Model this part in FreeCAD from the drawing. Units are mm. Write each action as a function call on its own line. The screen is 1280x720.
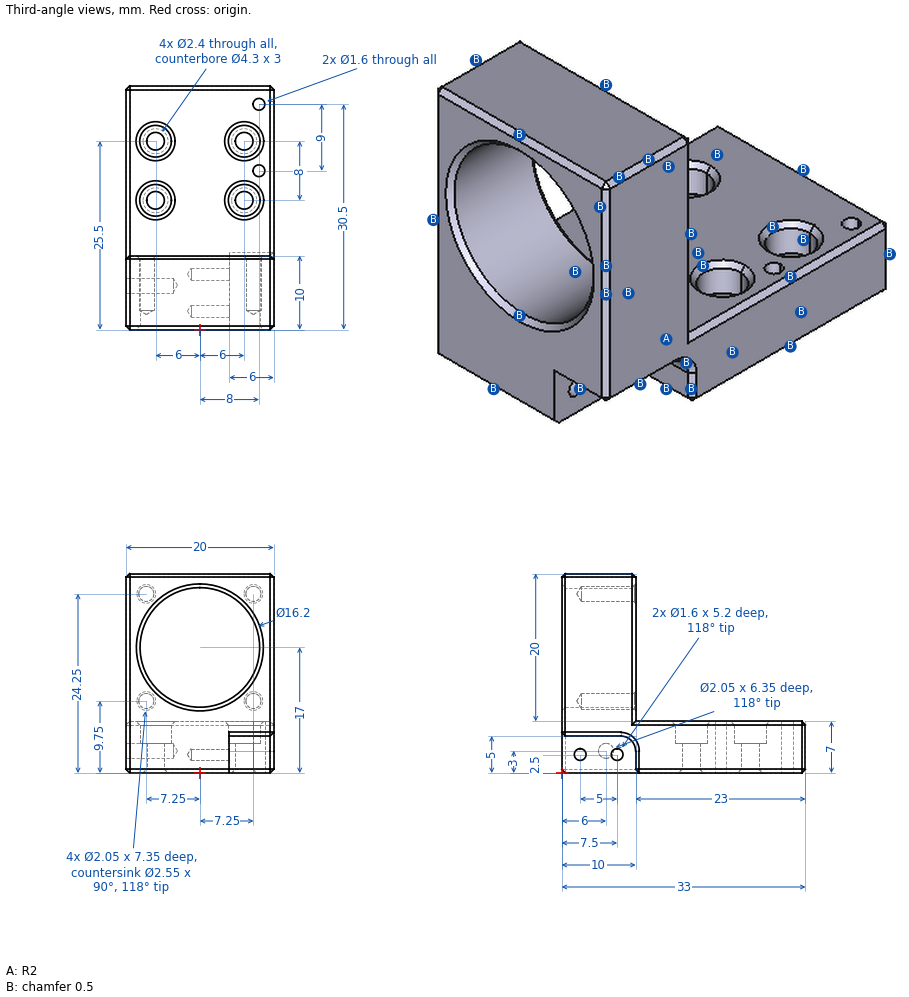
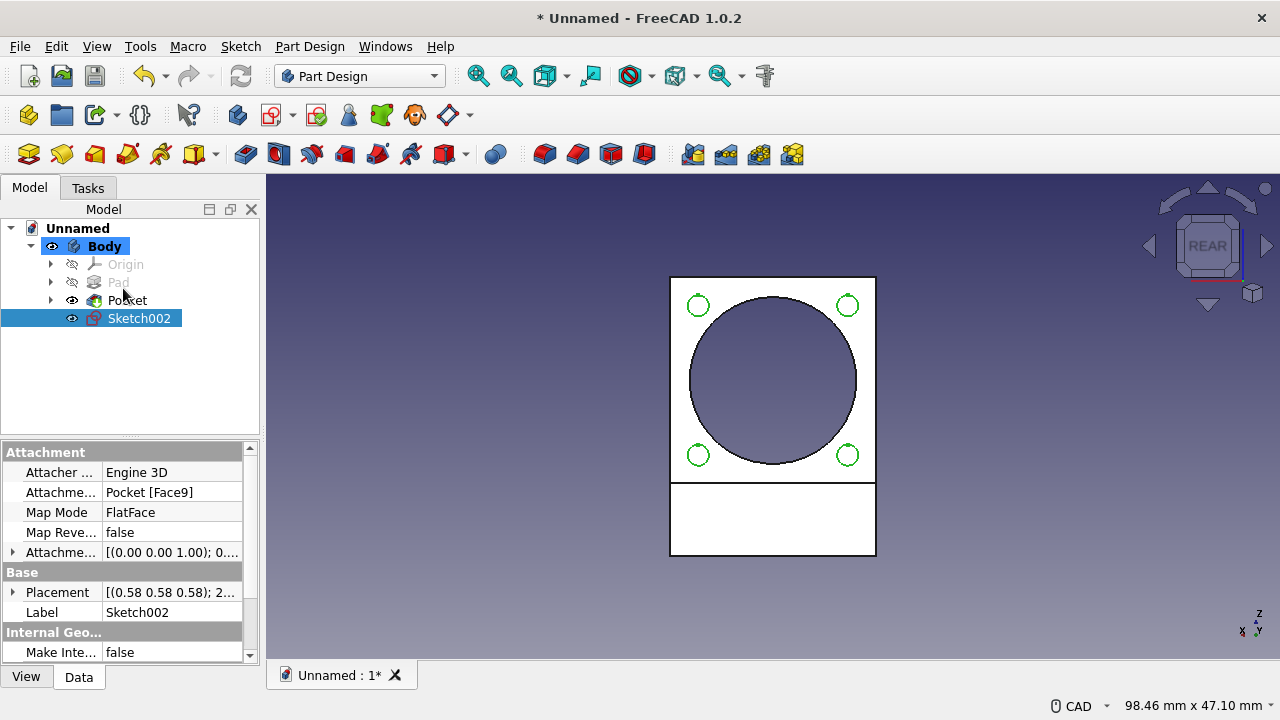
click(279, 154)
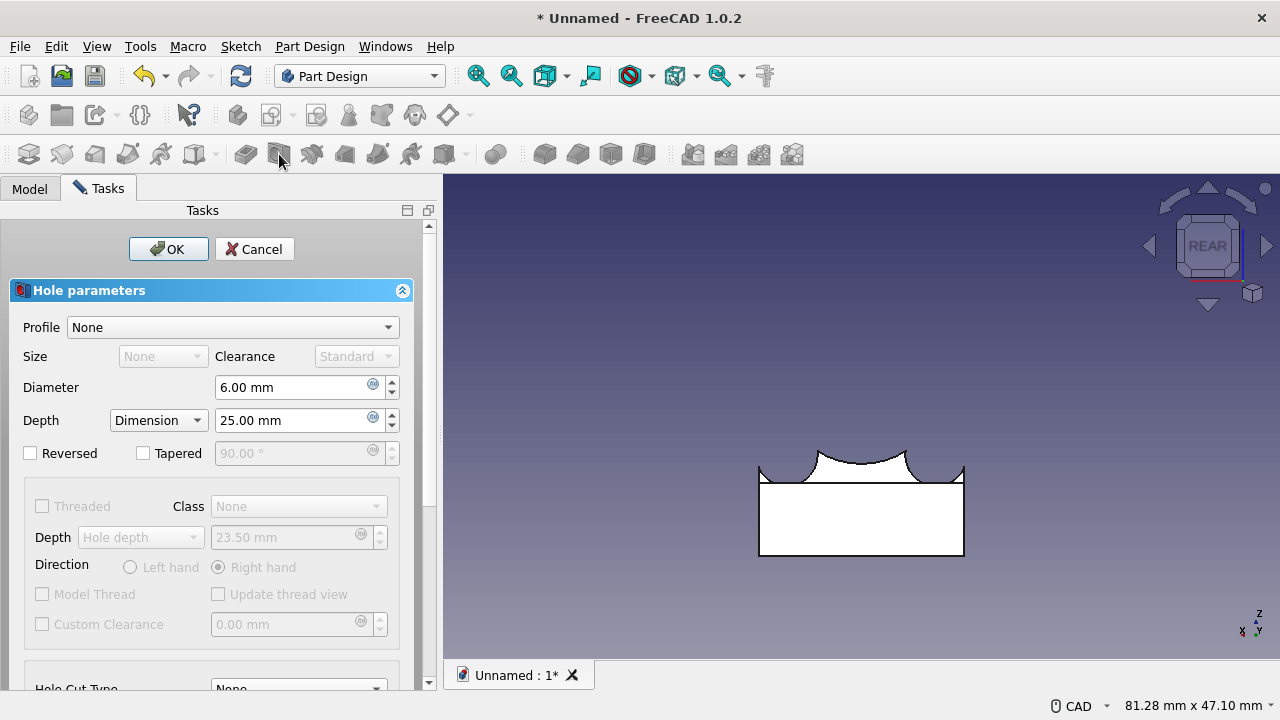
triple_click(300, 388)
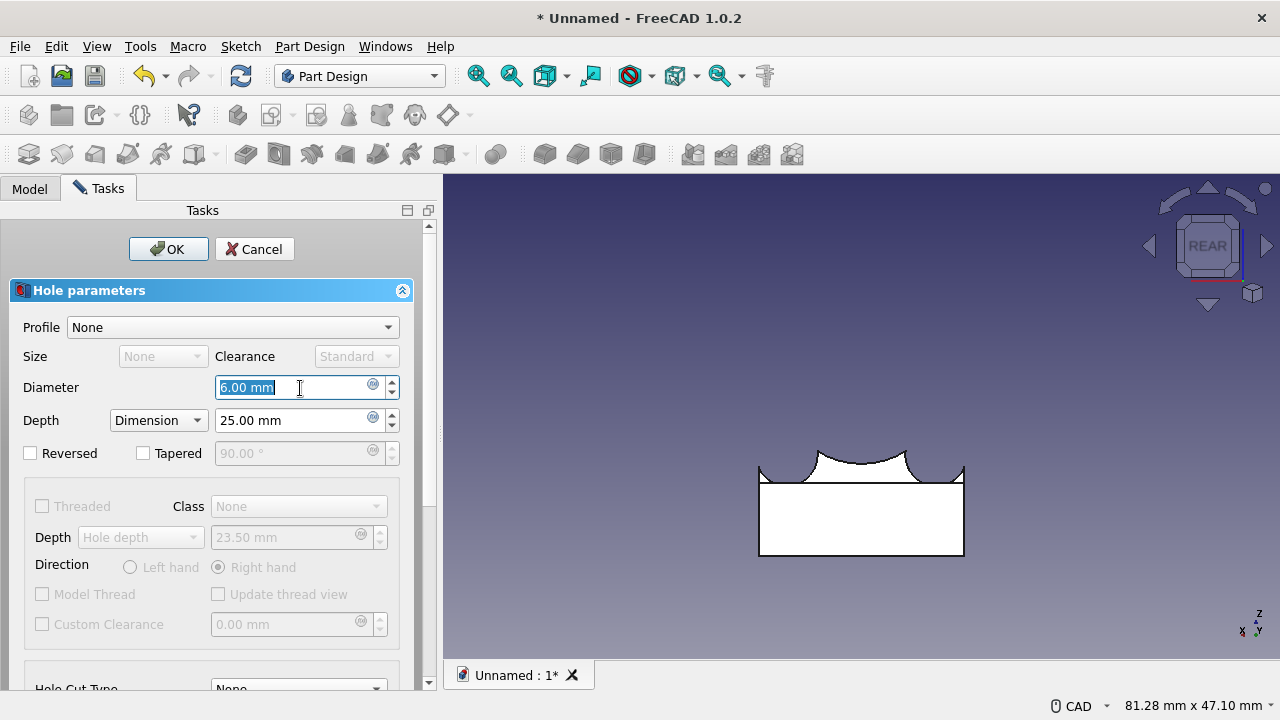
text(2.05)
key(Tab)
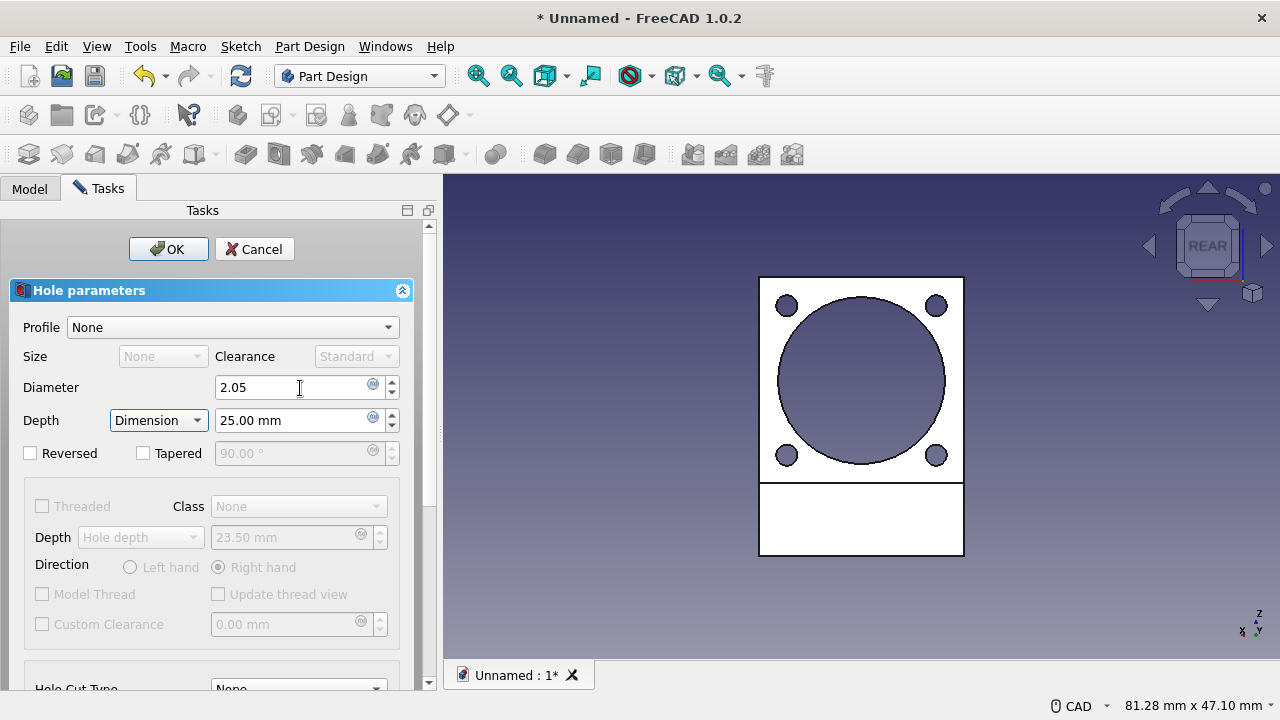
triple_click(300, 420)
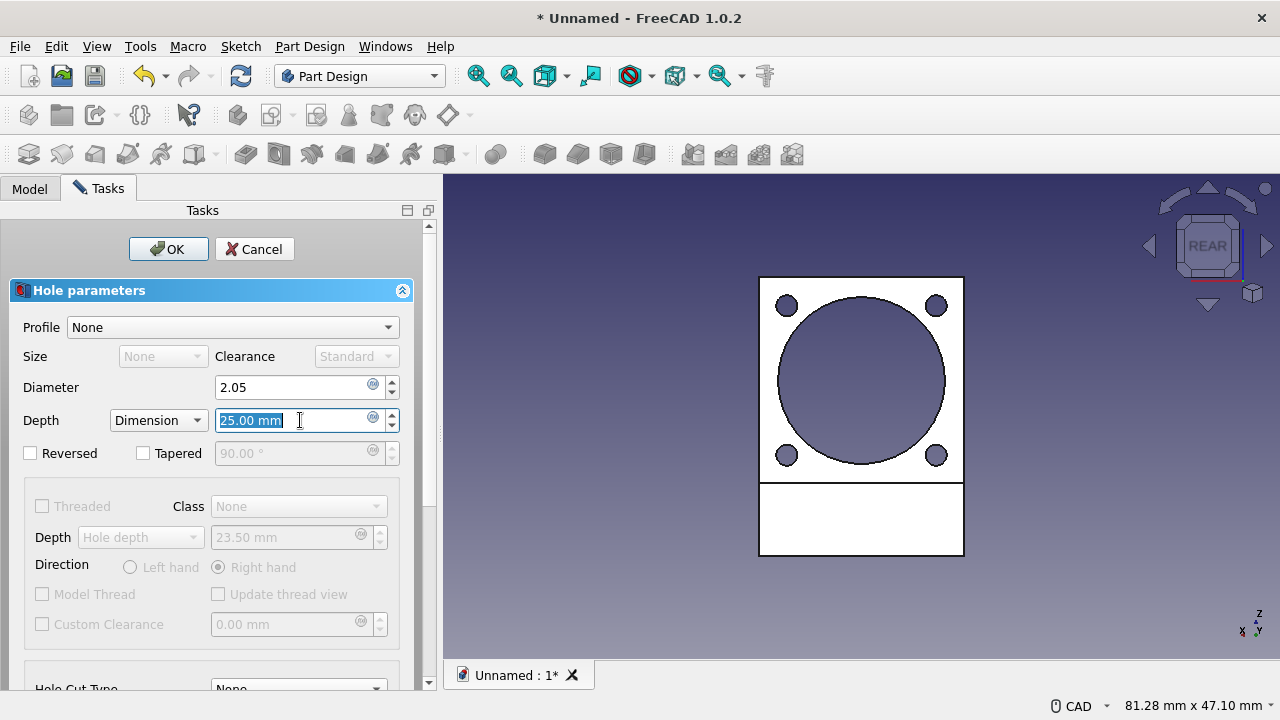
text(7.35)
key(Tab)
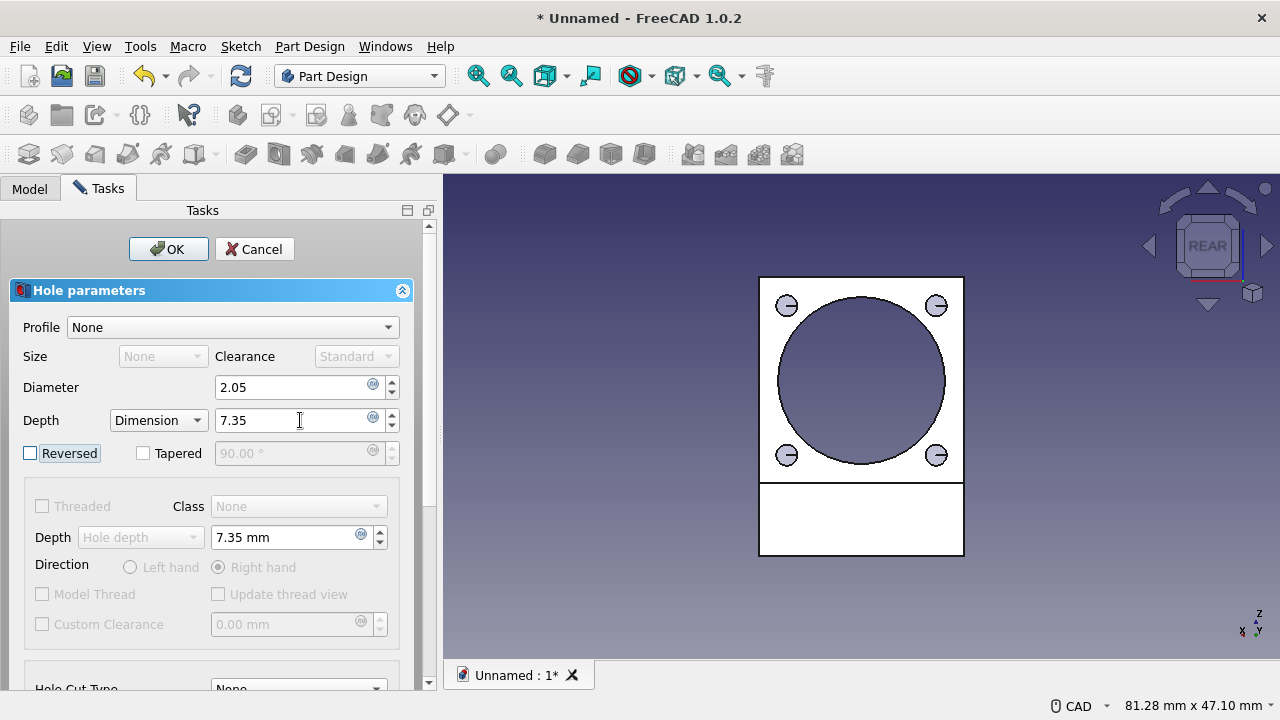
scroll(429, 455, down, 2)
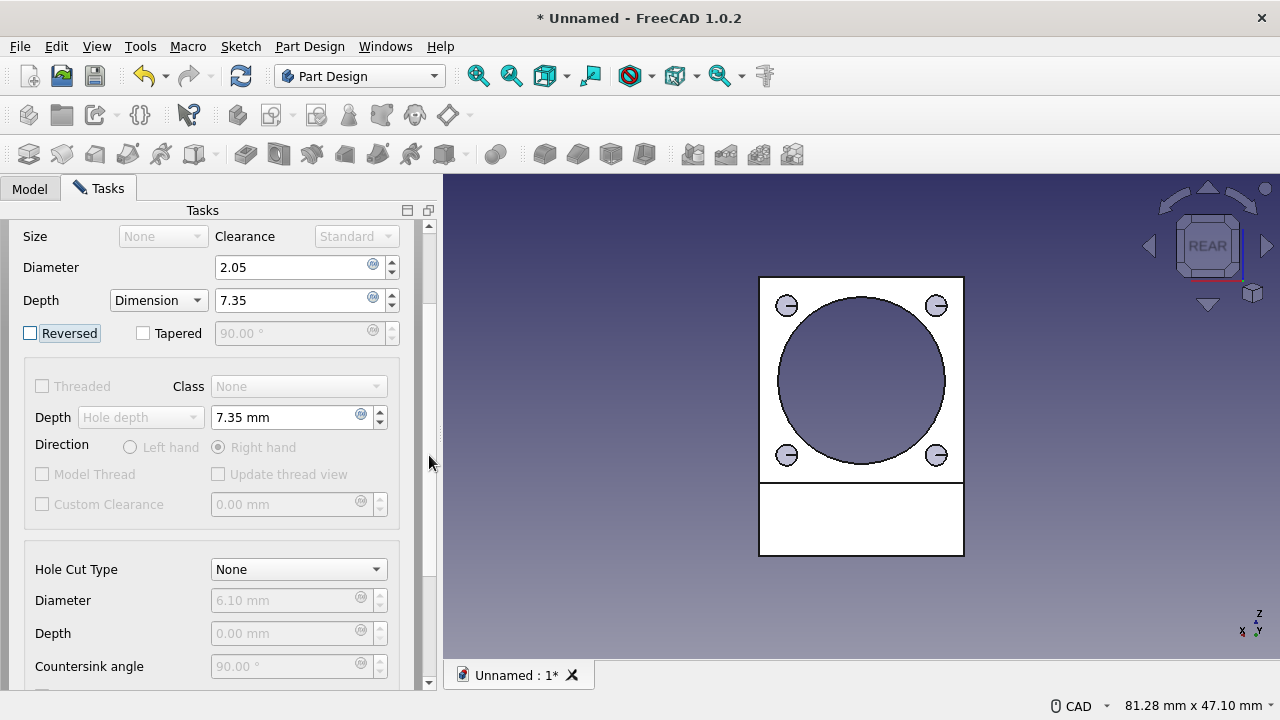
click(300, 570)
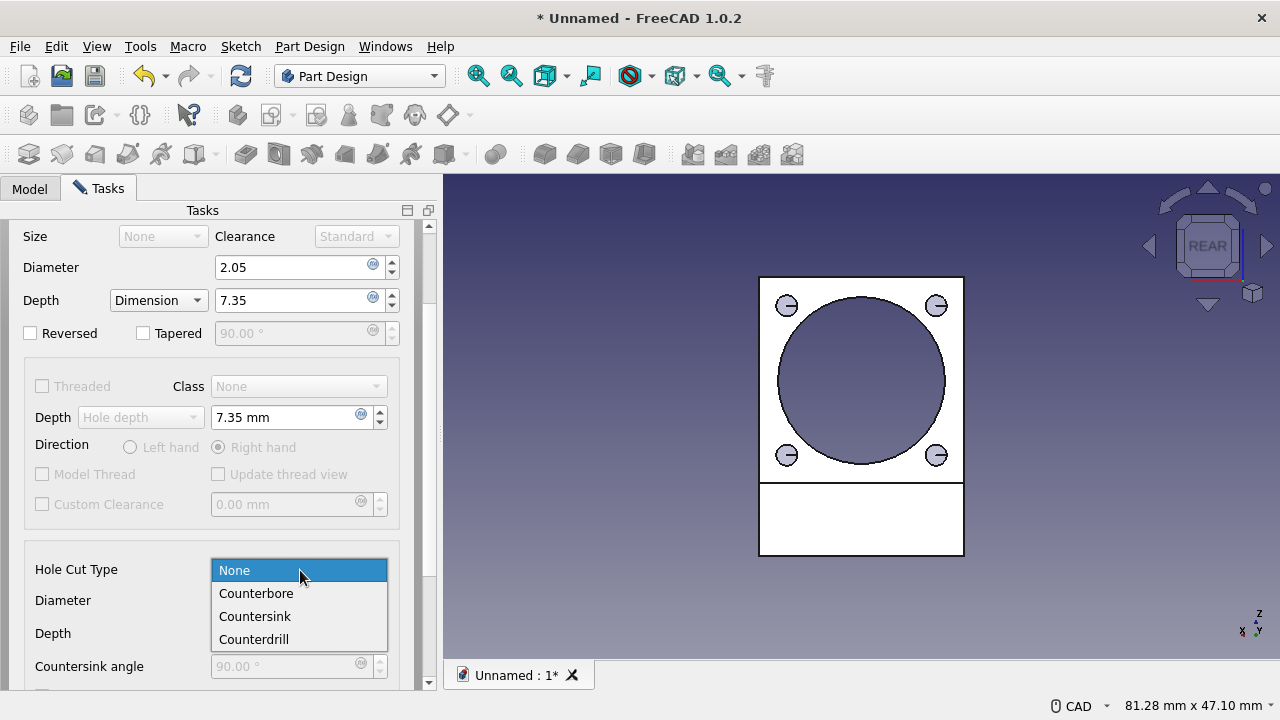
click(298, 616)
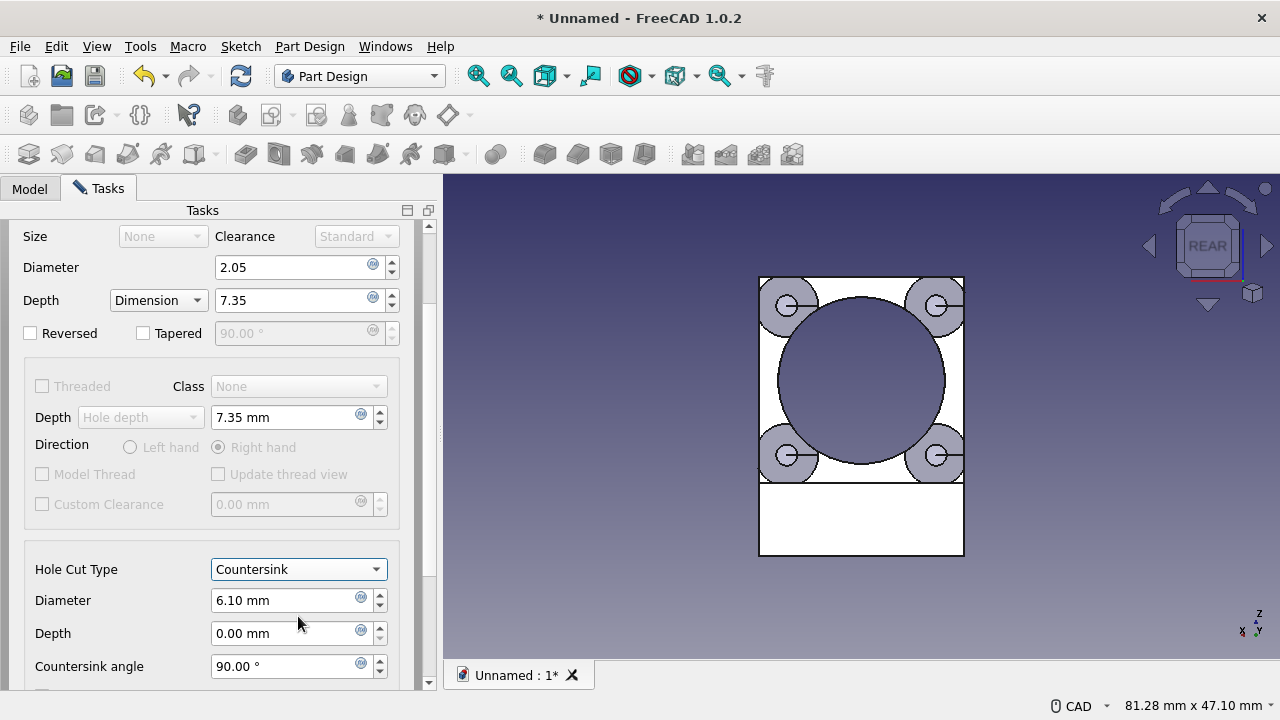
triple_click(292, 600)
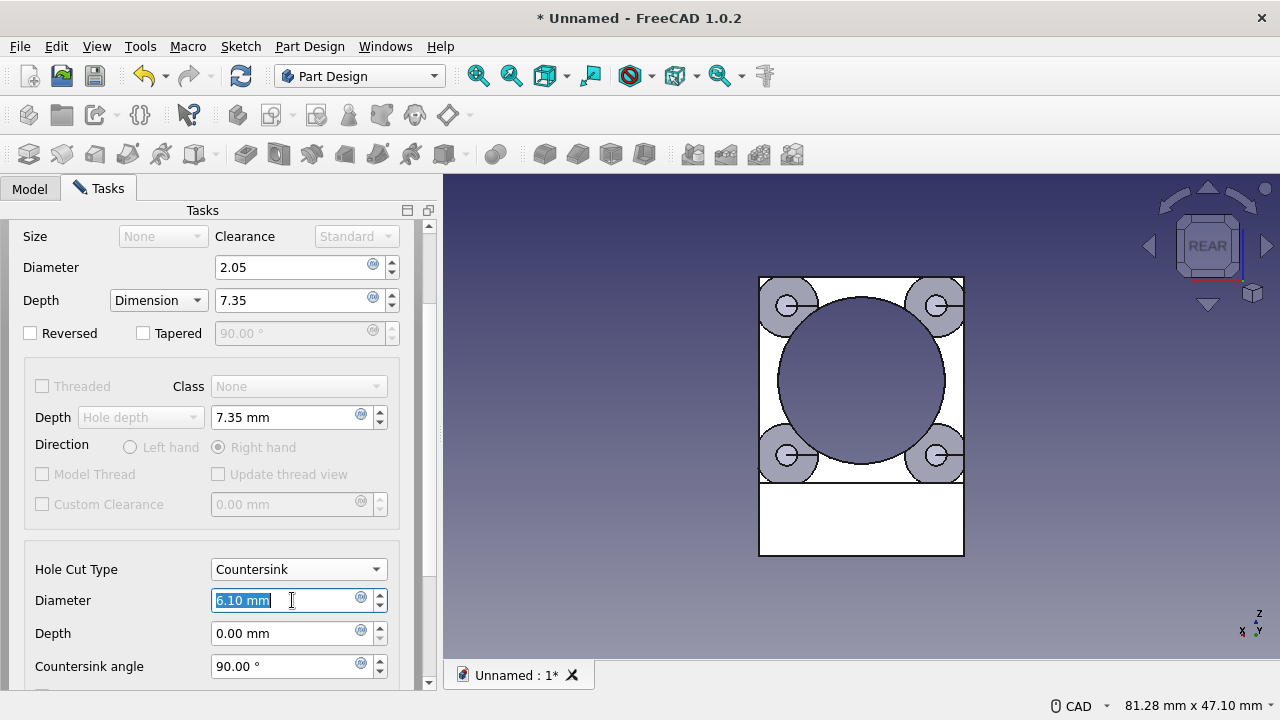
text(2.55)
key(Tab)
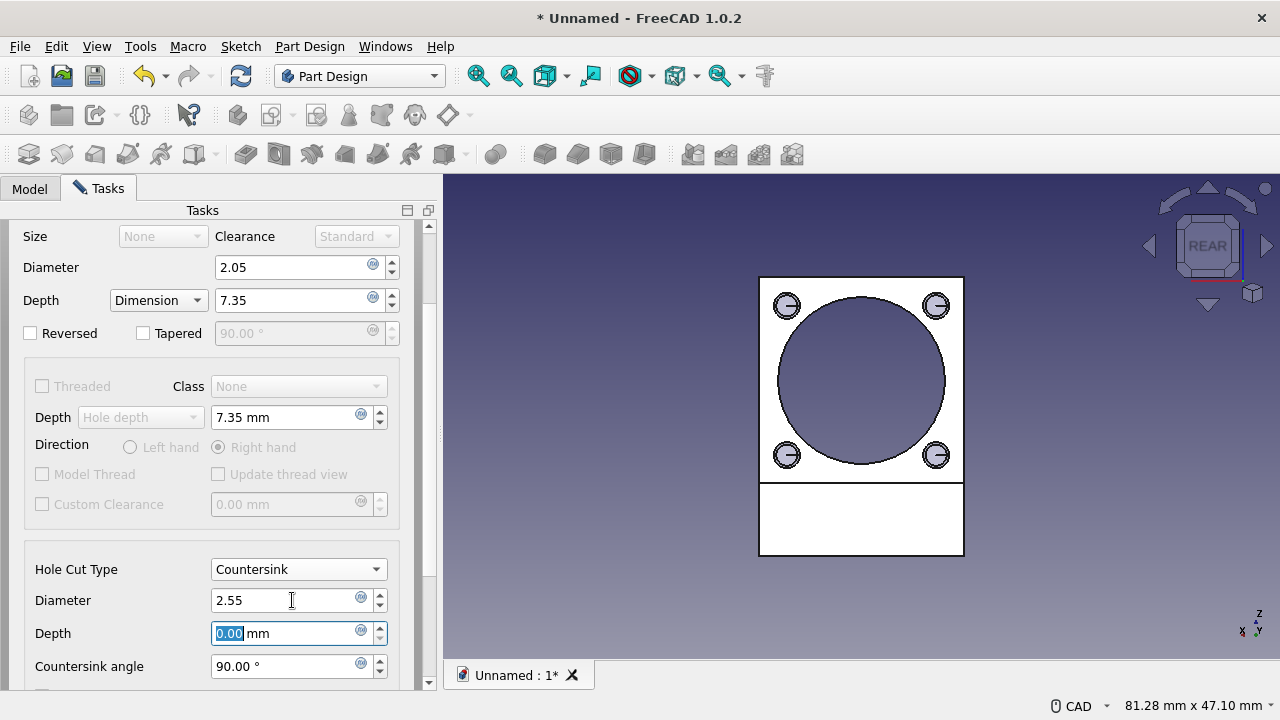
scroll(429, 455, up, 3)